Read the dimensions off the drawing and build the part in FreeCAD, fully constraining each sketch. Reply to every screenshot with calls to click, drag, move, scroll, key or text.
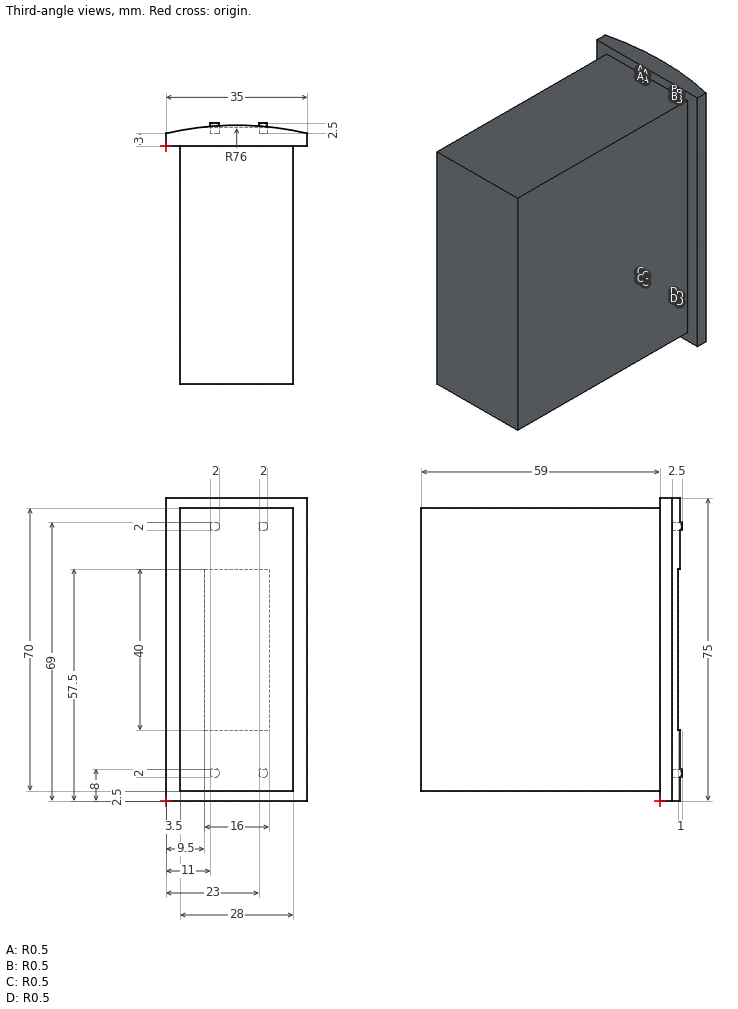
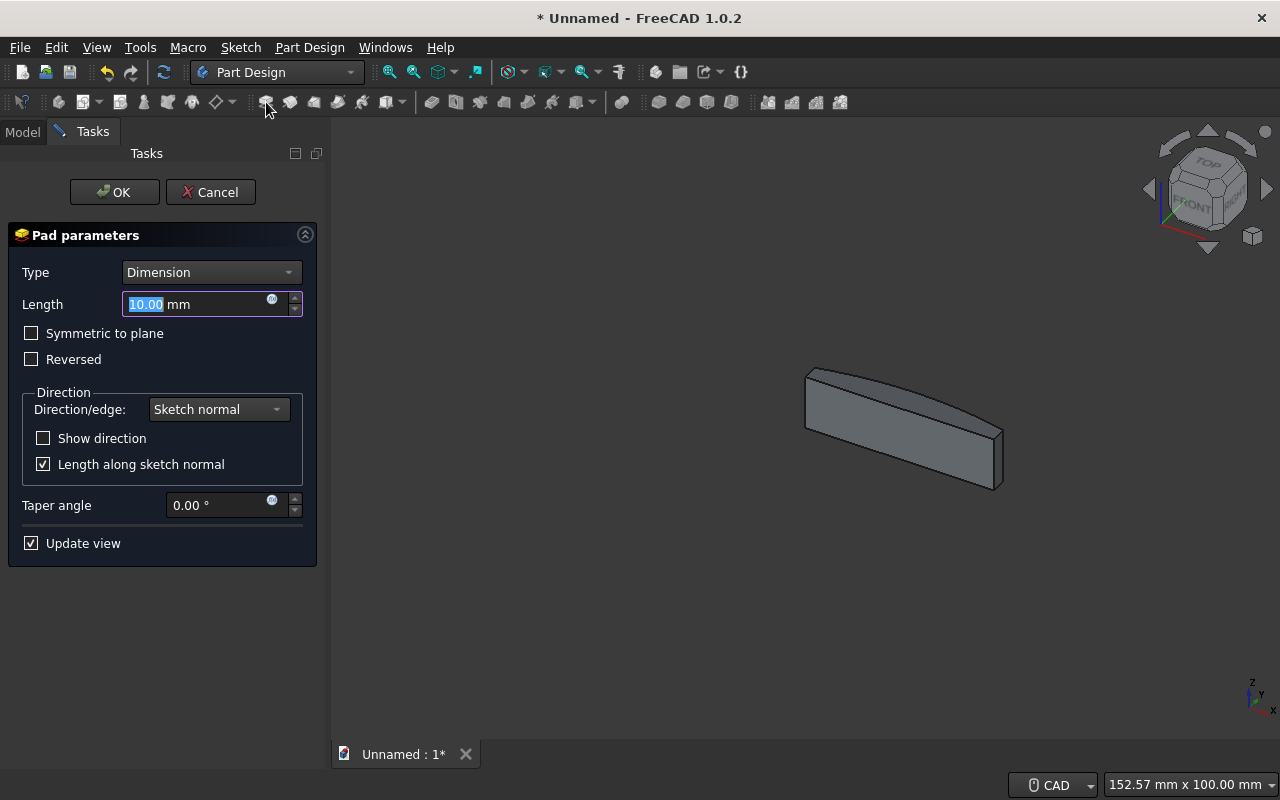
text(75)
key(Tab)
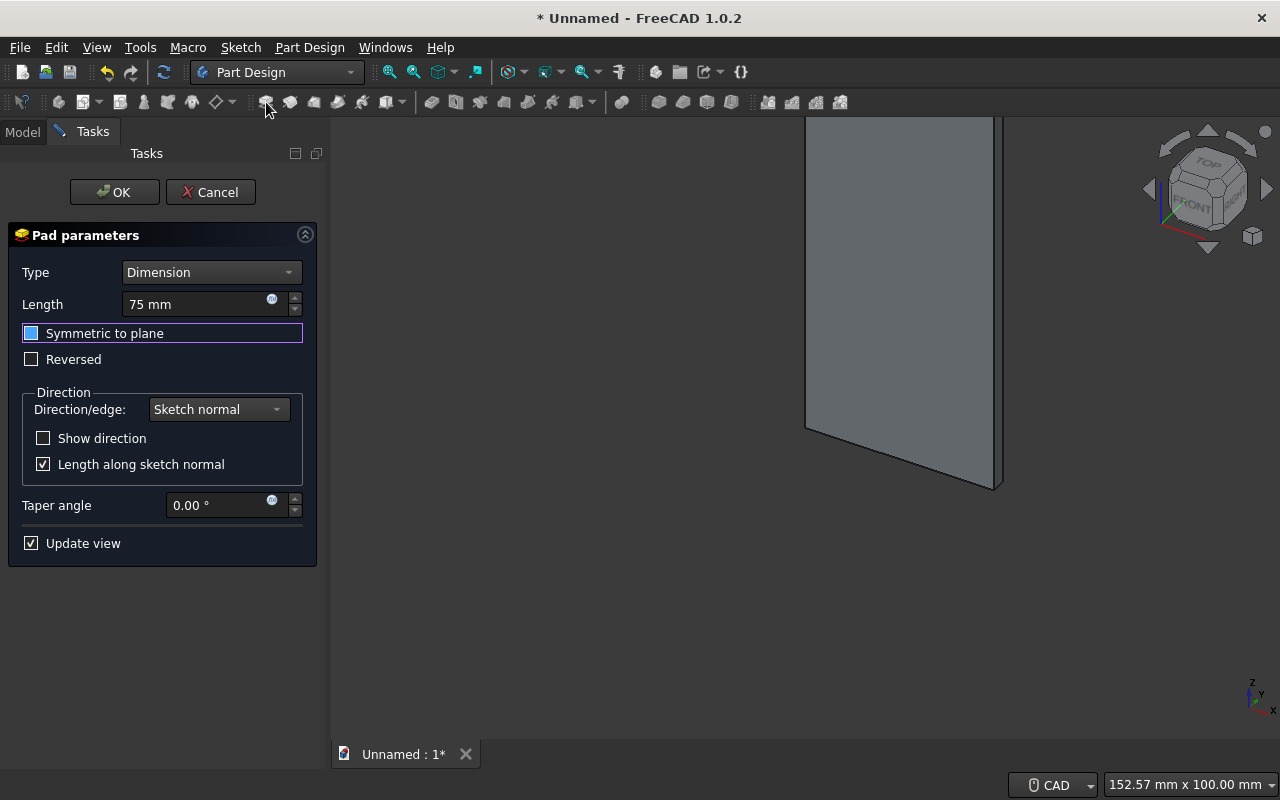
click(115, 192)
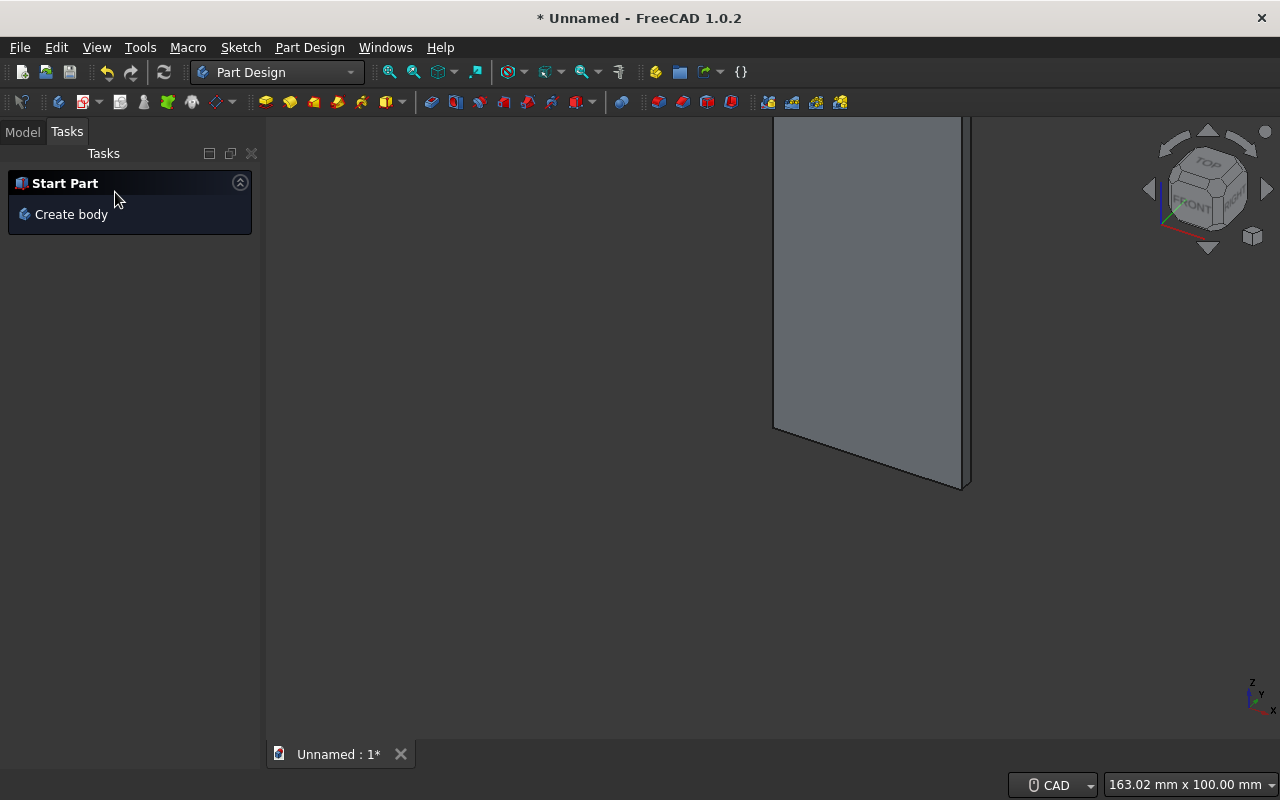
key(v)
key(f)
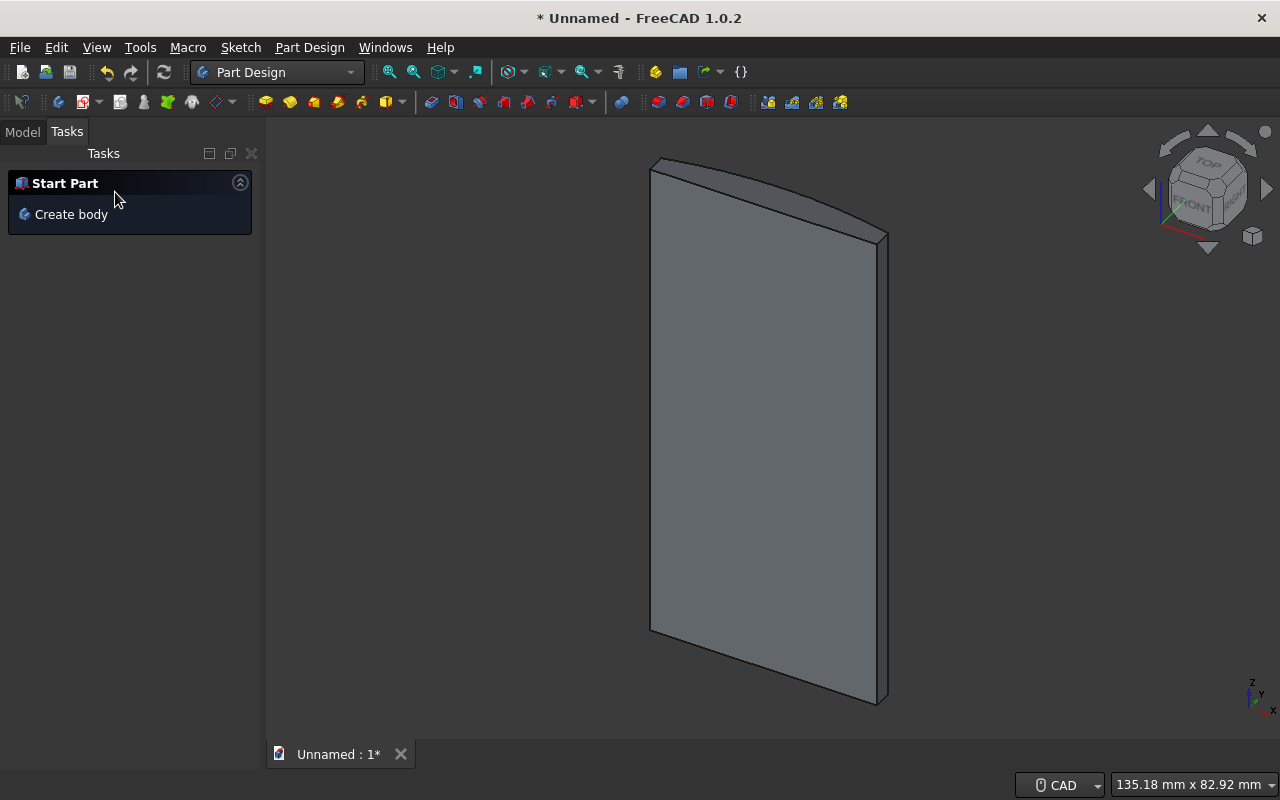
click(23, 131)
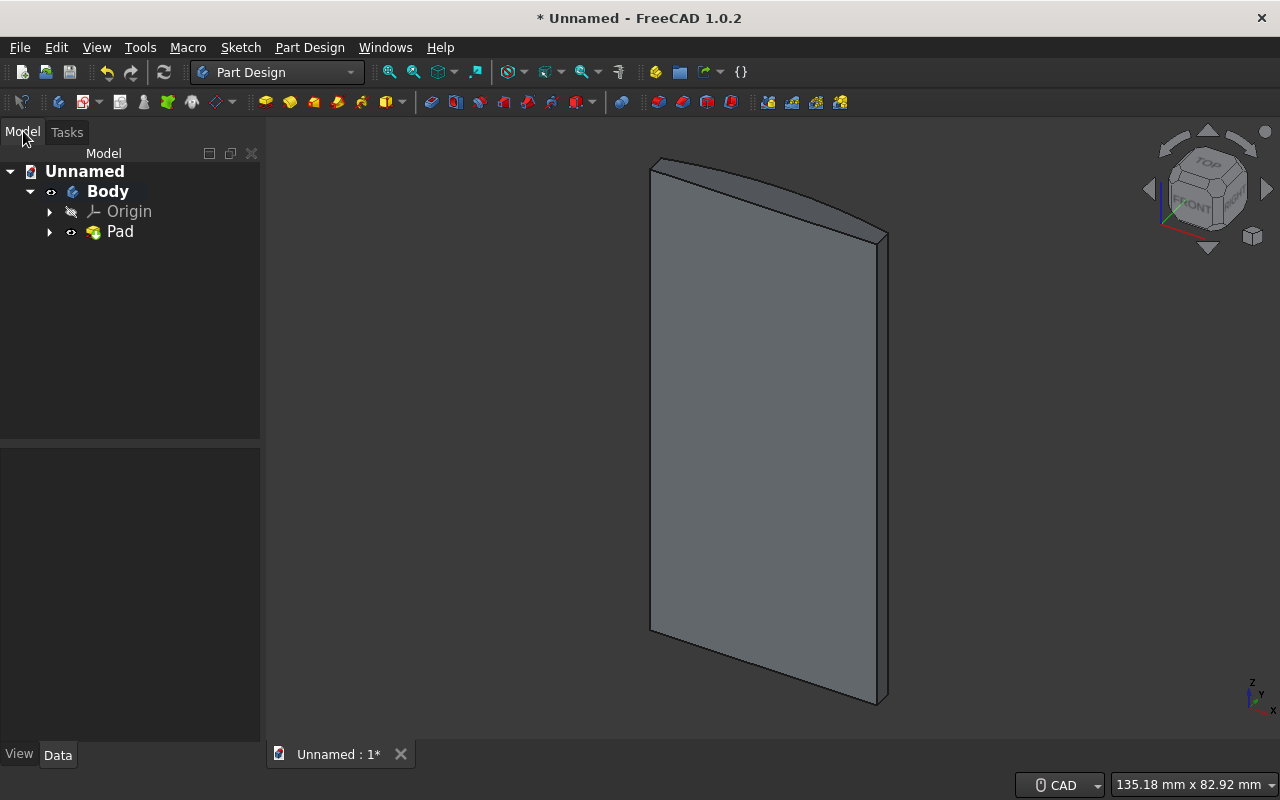
click(50, 212)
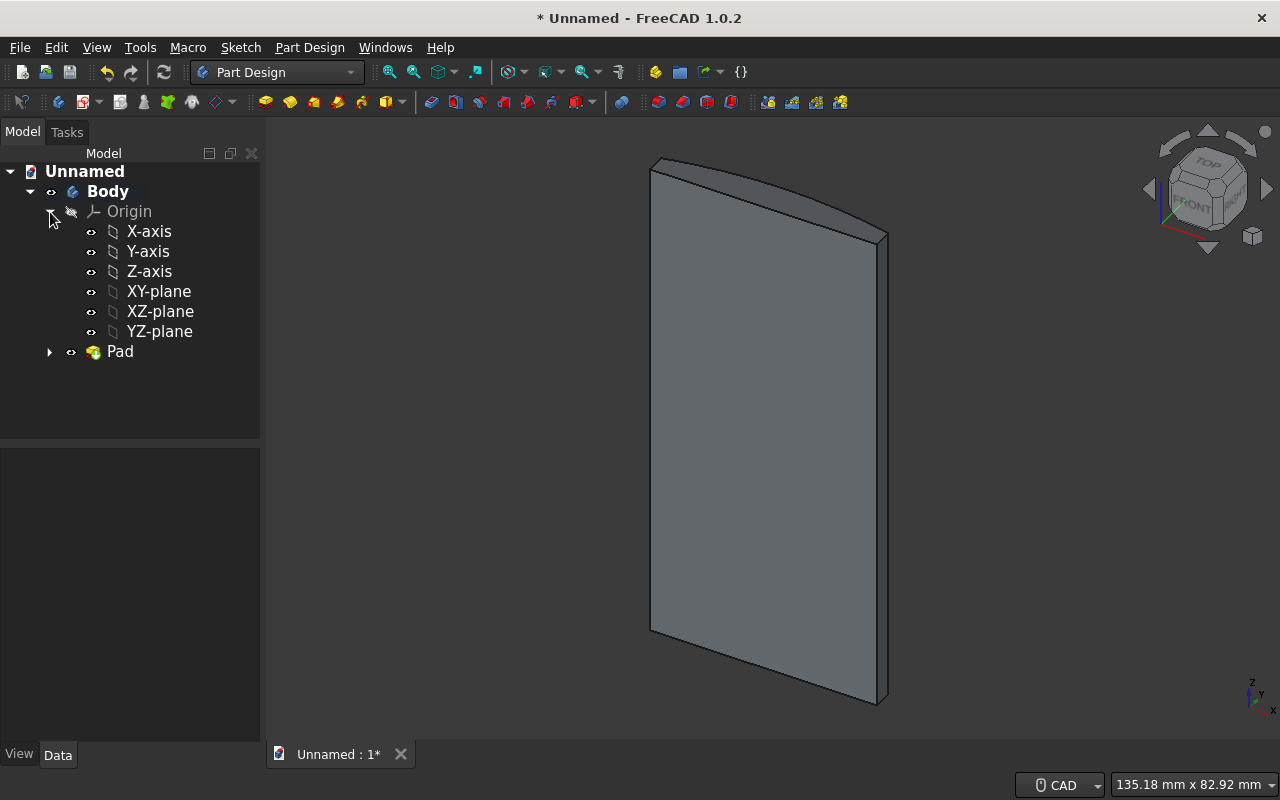
click(136, 312)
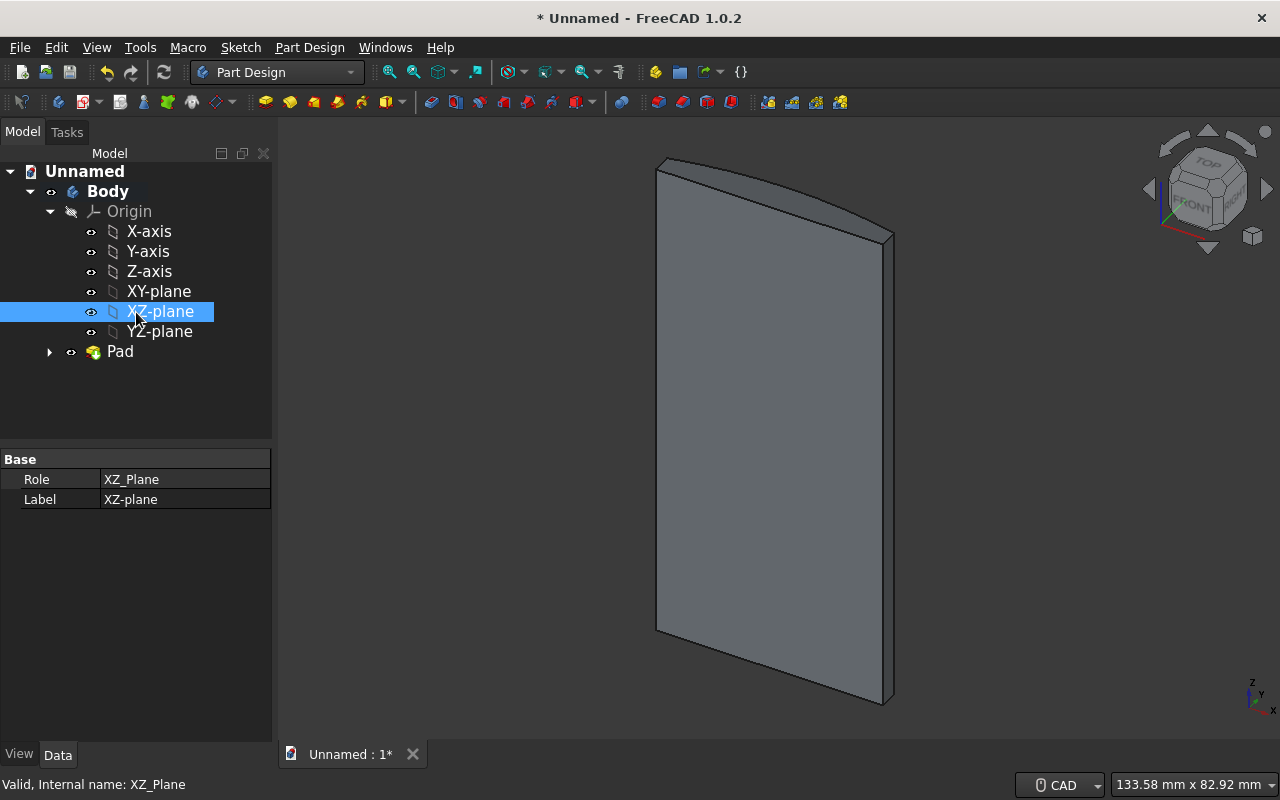
click(216, 102)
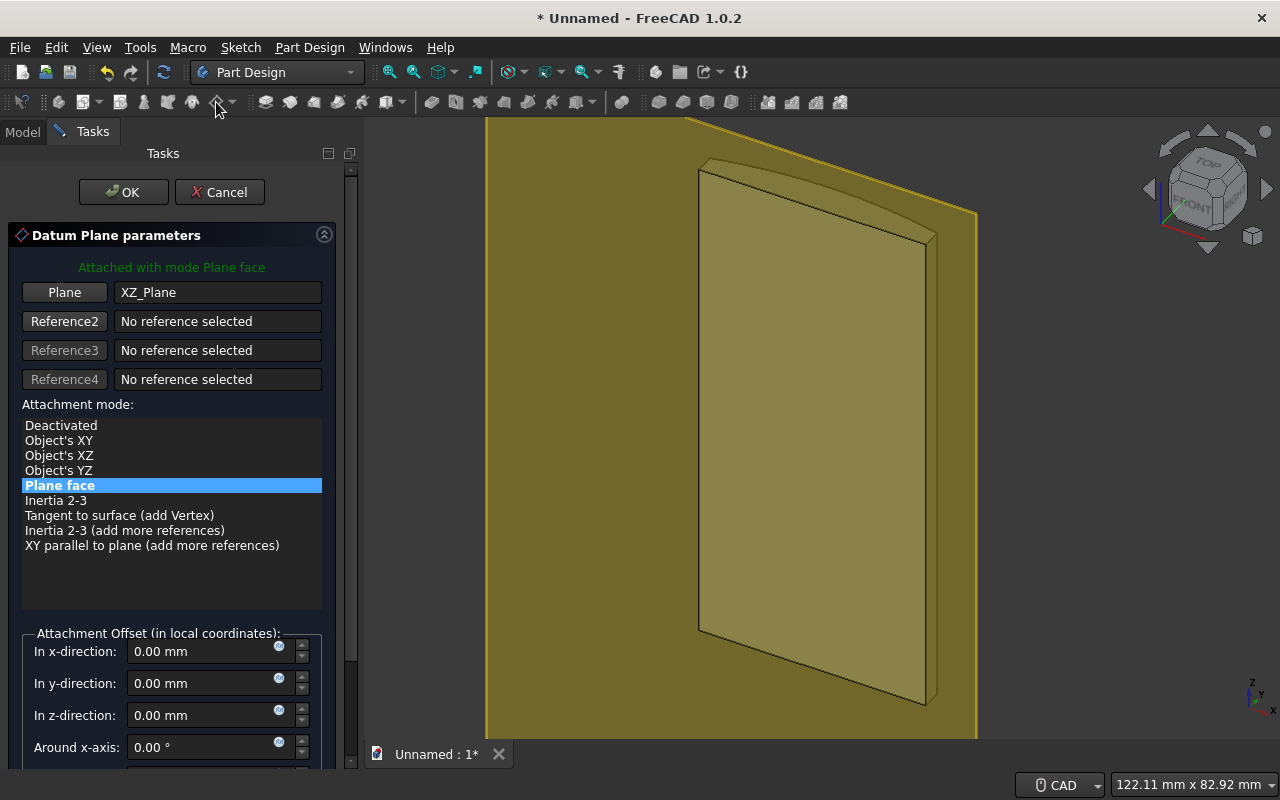
triple_click(210, 715)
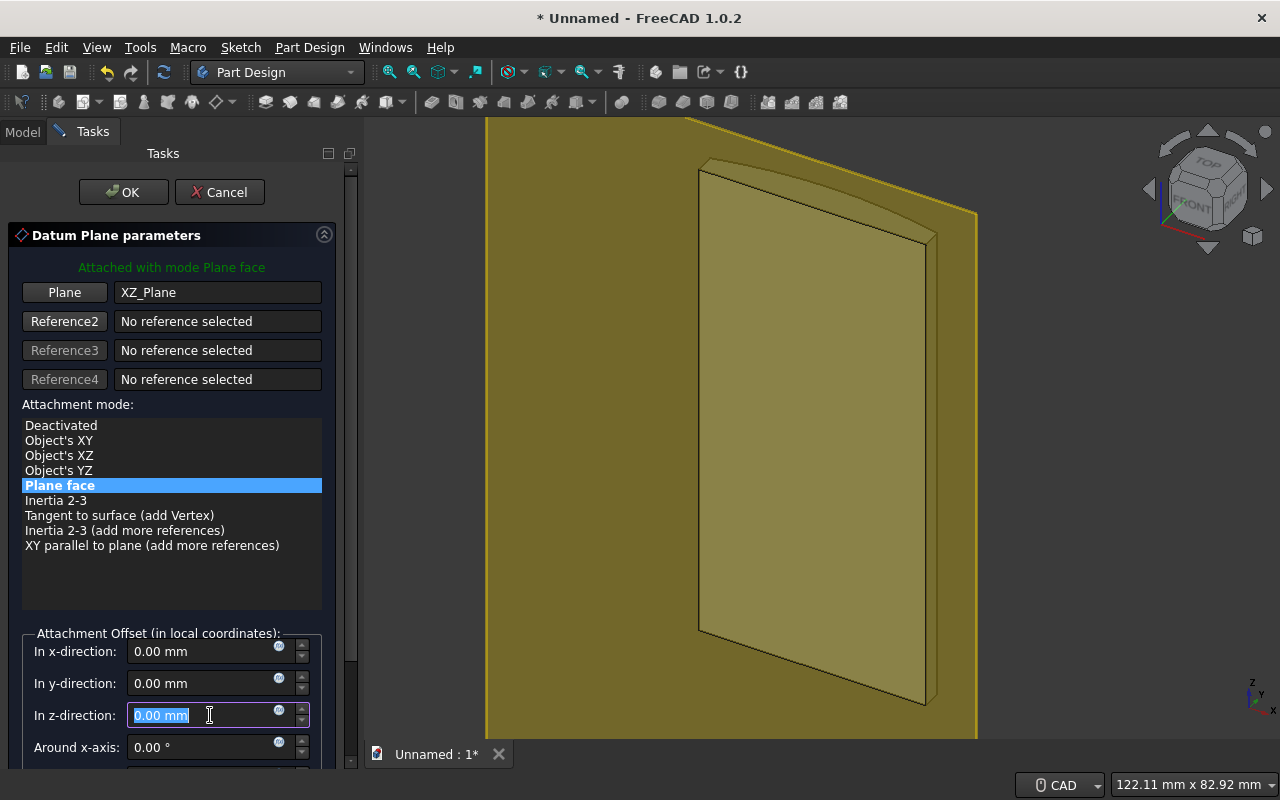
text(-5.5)
key(Tab)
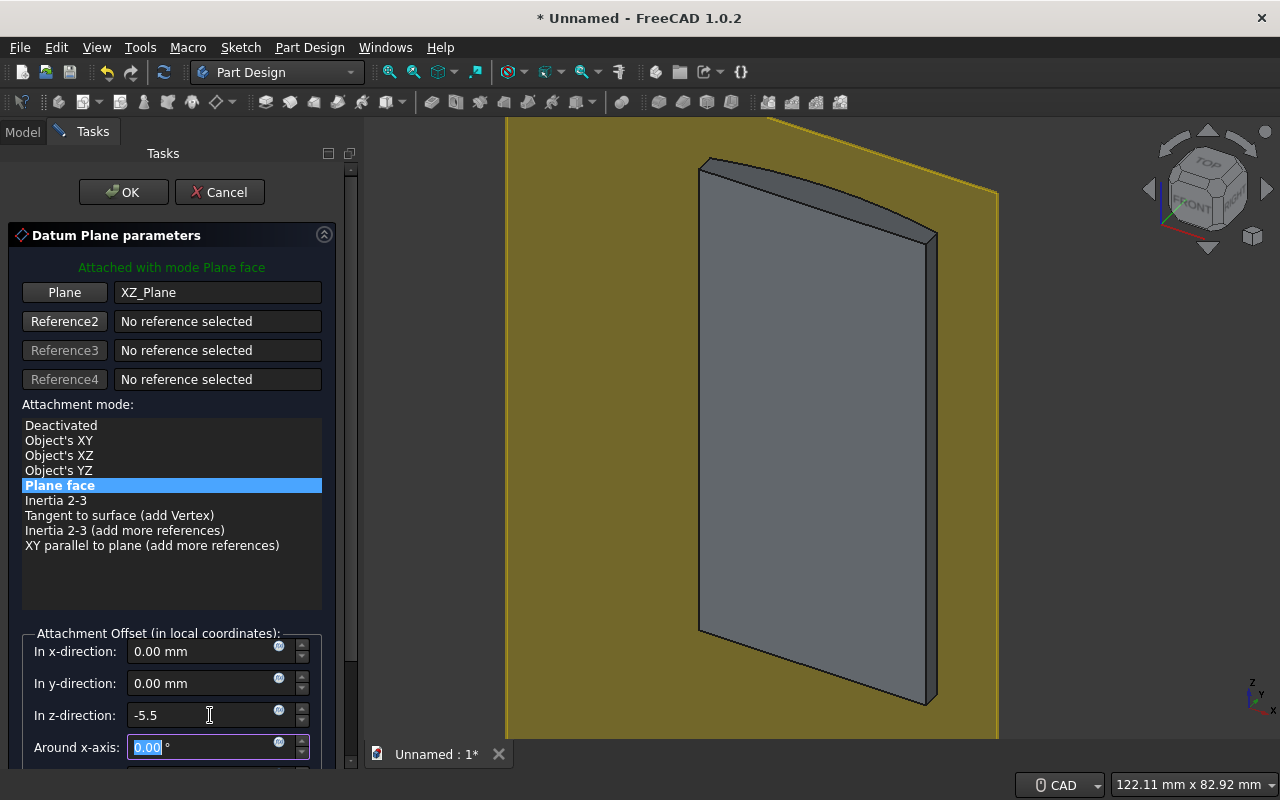
click(124, 192)